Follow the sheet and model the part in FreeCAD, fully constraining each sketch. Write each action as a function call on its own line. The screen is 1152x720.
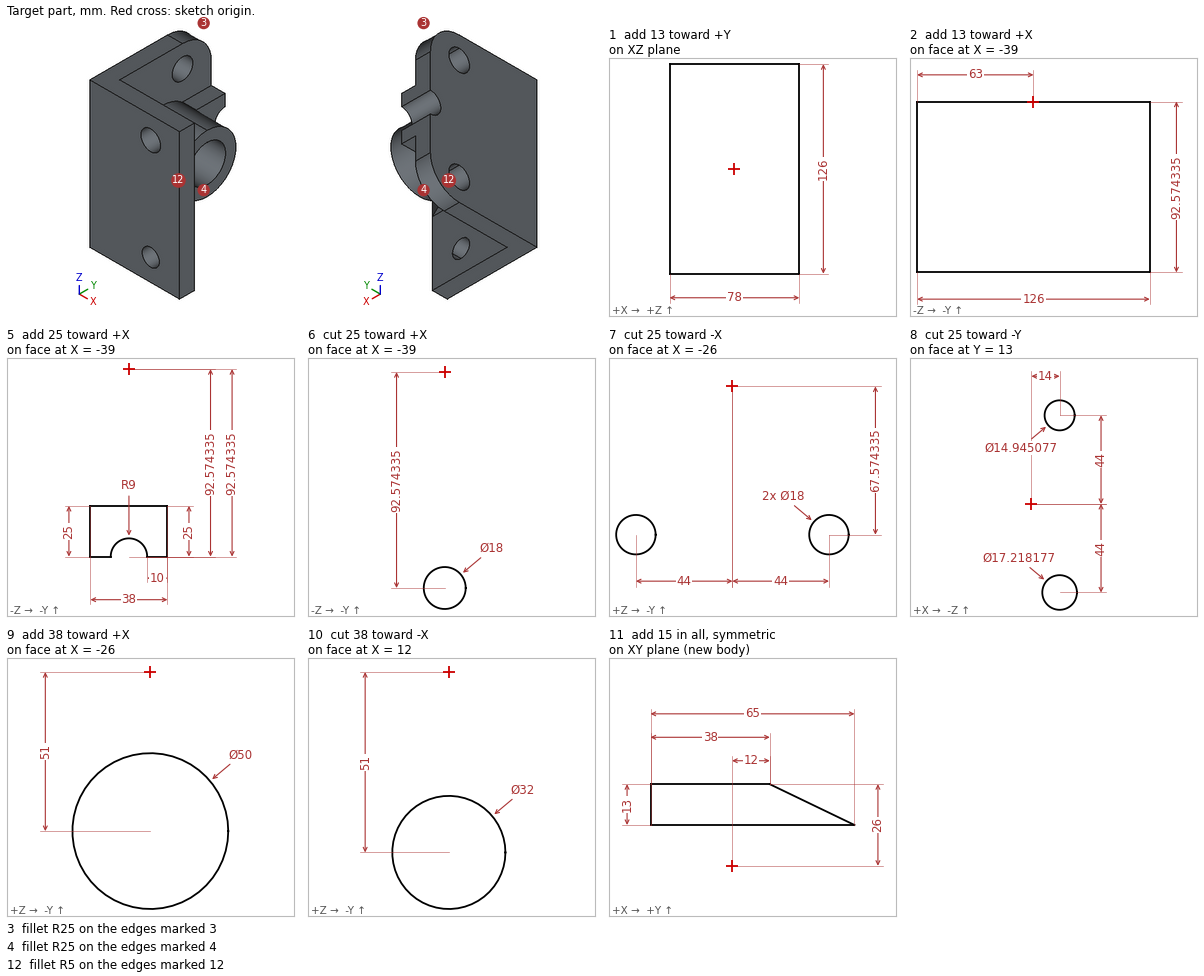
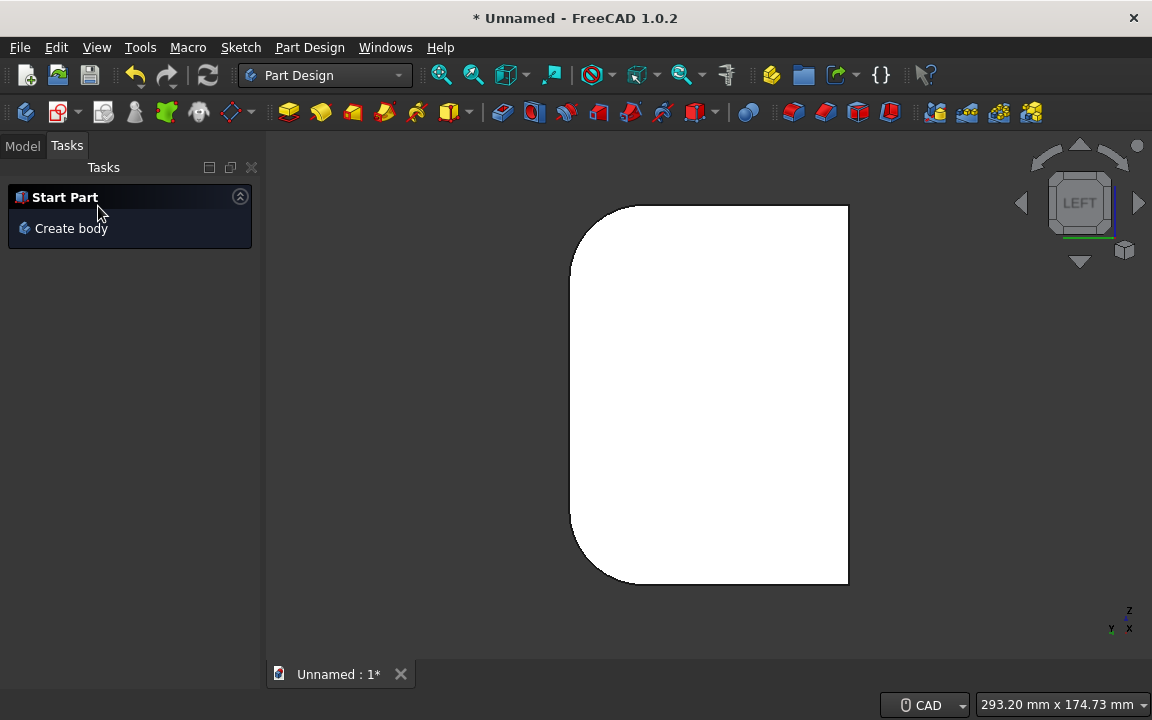
click(709, 394)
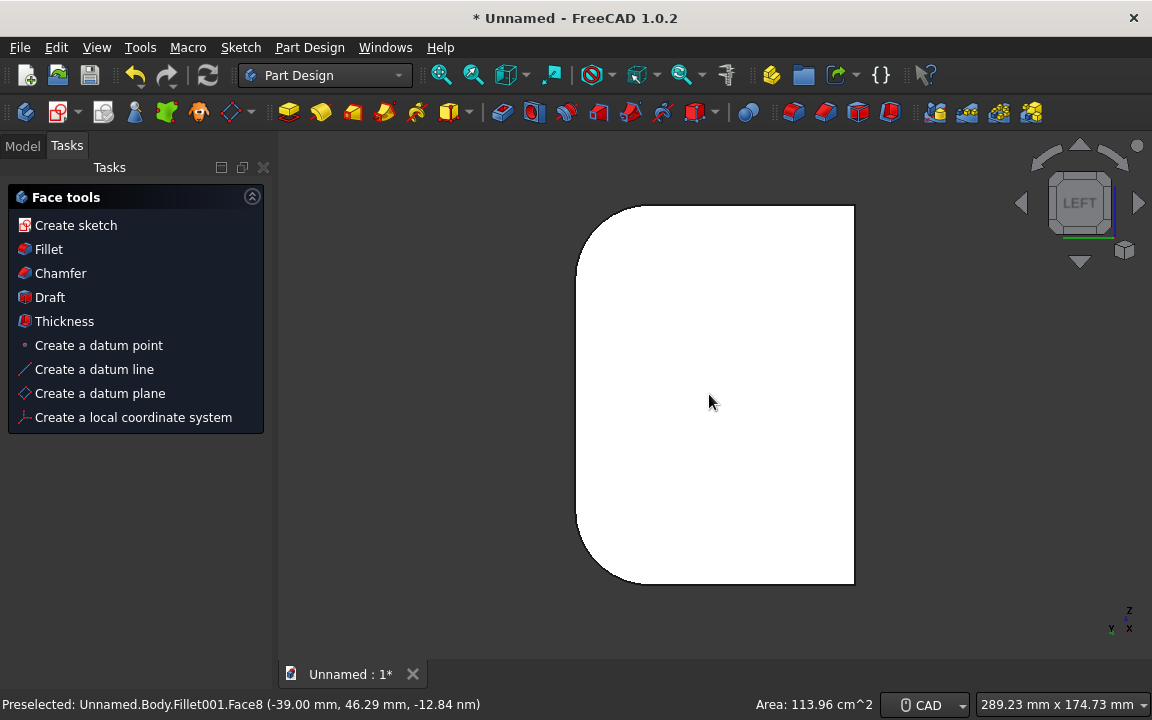
click(58, 112)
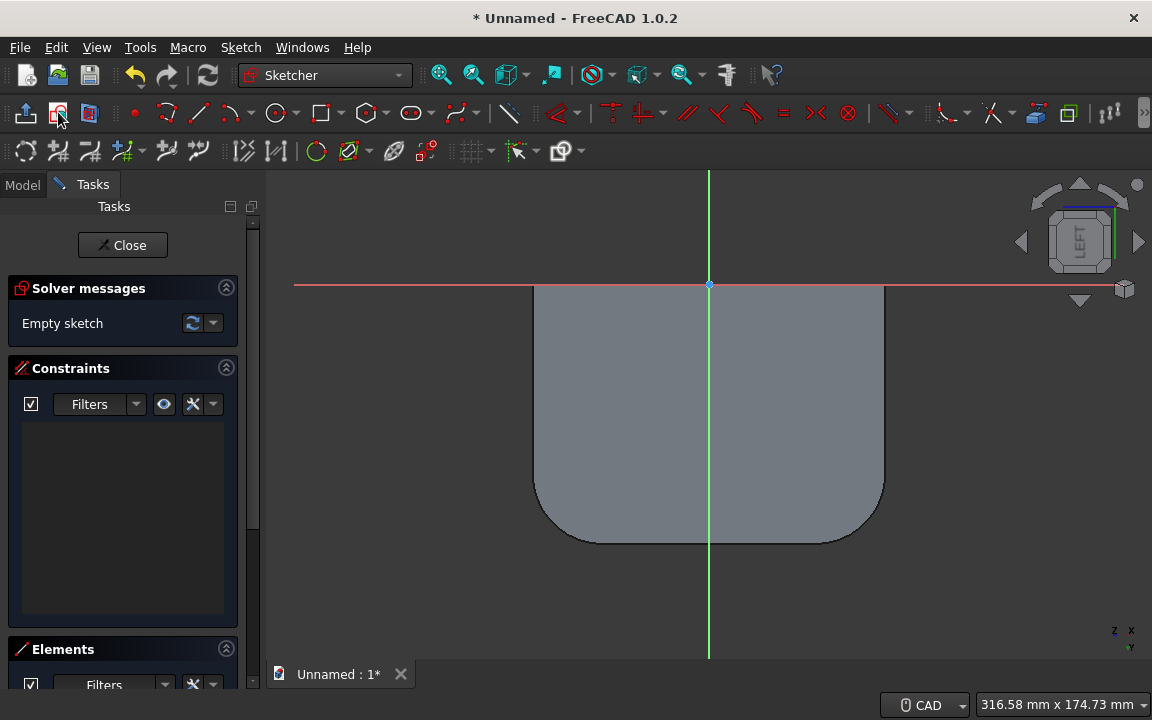
click(168, 114)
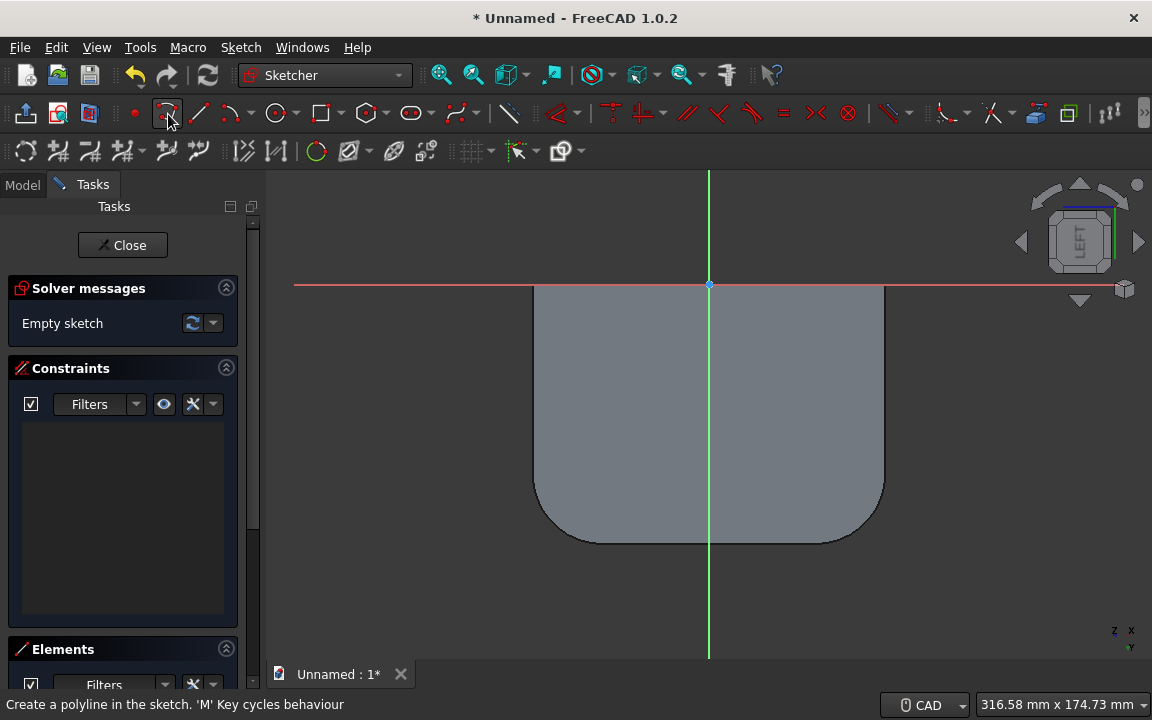
click(734, 544)
click(762, 544)
click(762, 474)
click(656, 474)
click(656, 544)
click(684, 544)
right_click(684, 544)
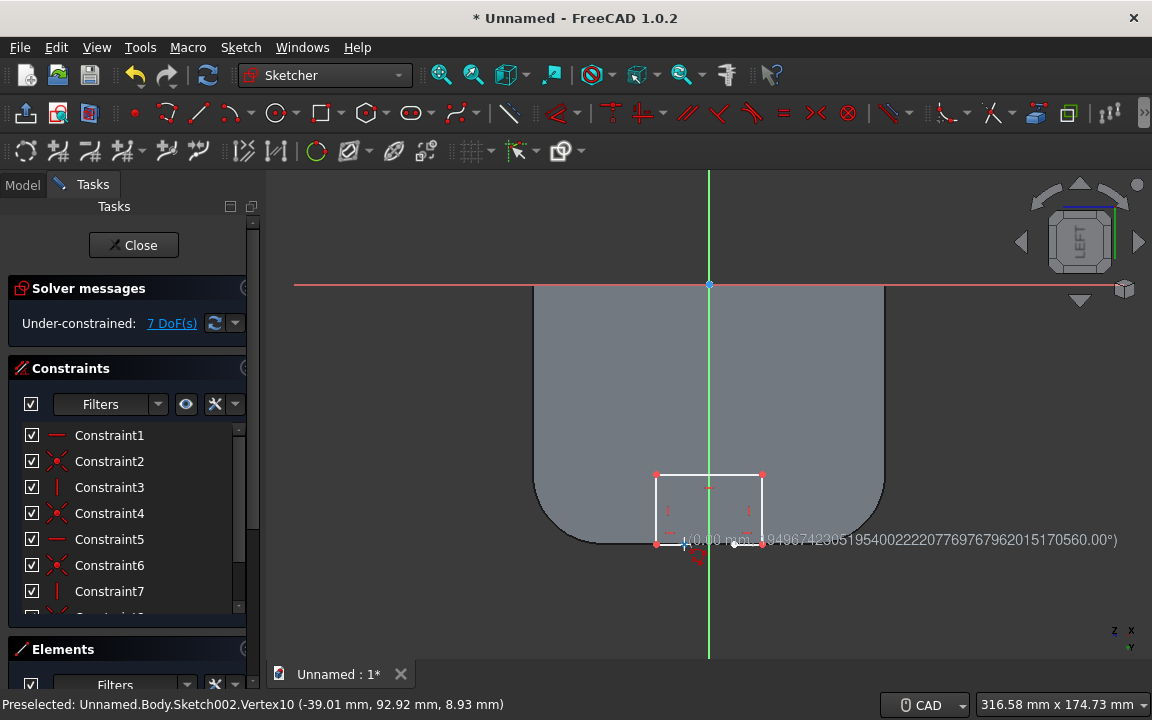
key(g)
key(3)
key(a)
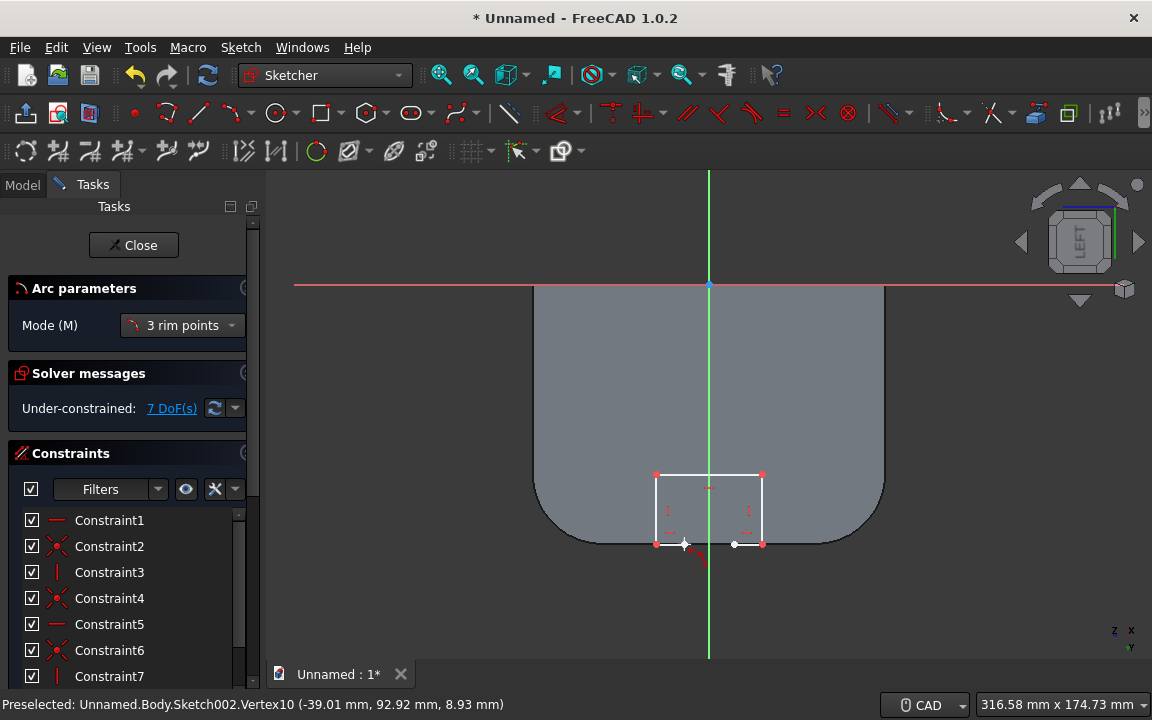
click(684, 545)
click(734, 545)
click(724, 524)
key(Escape)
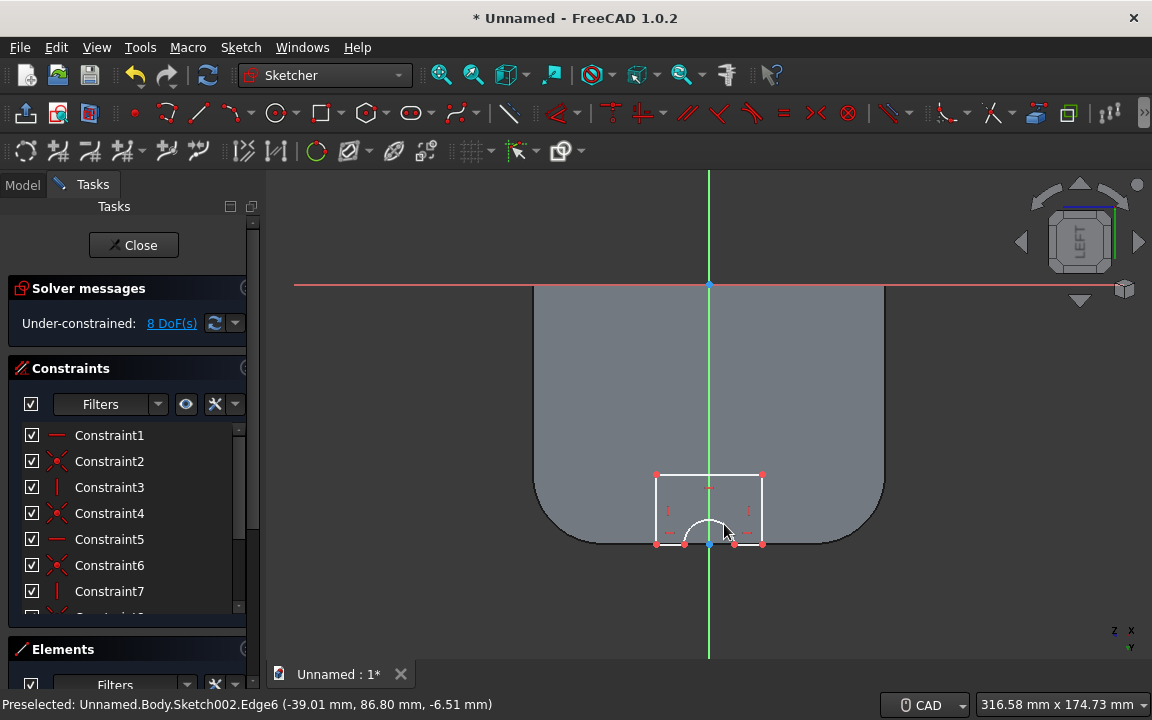
click(709, 545)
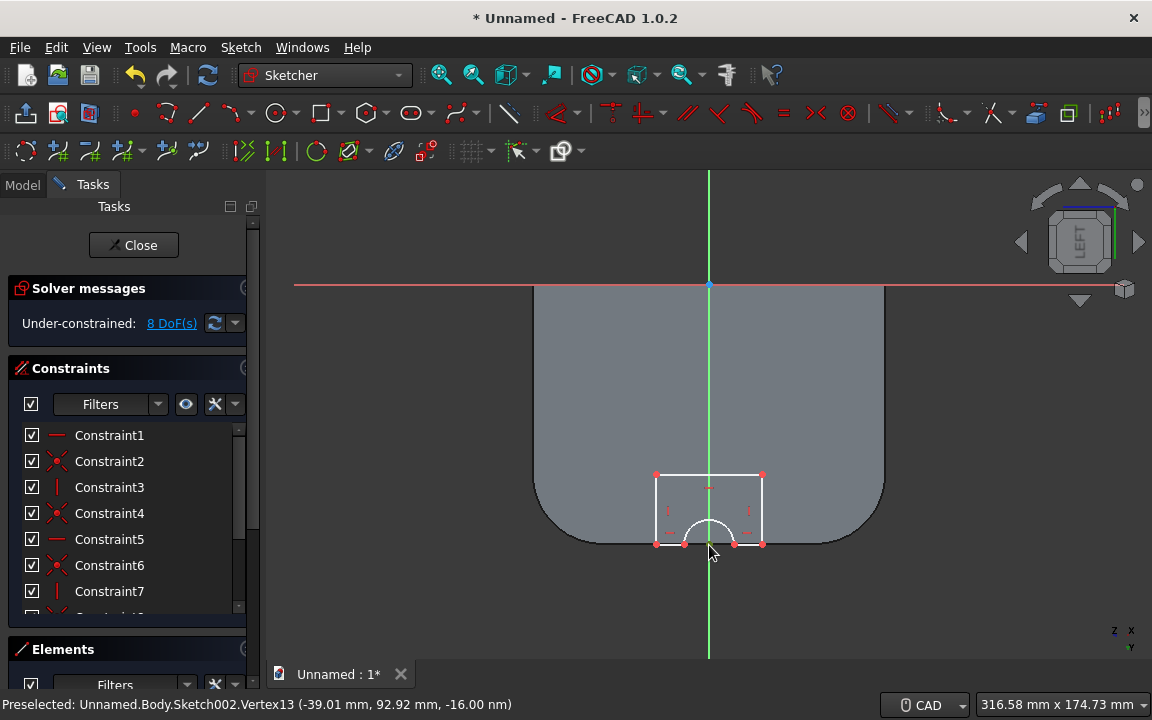
click(709, 600)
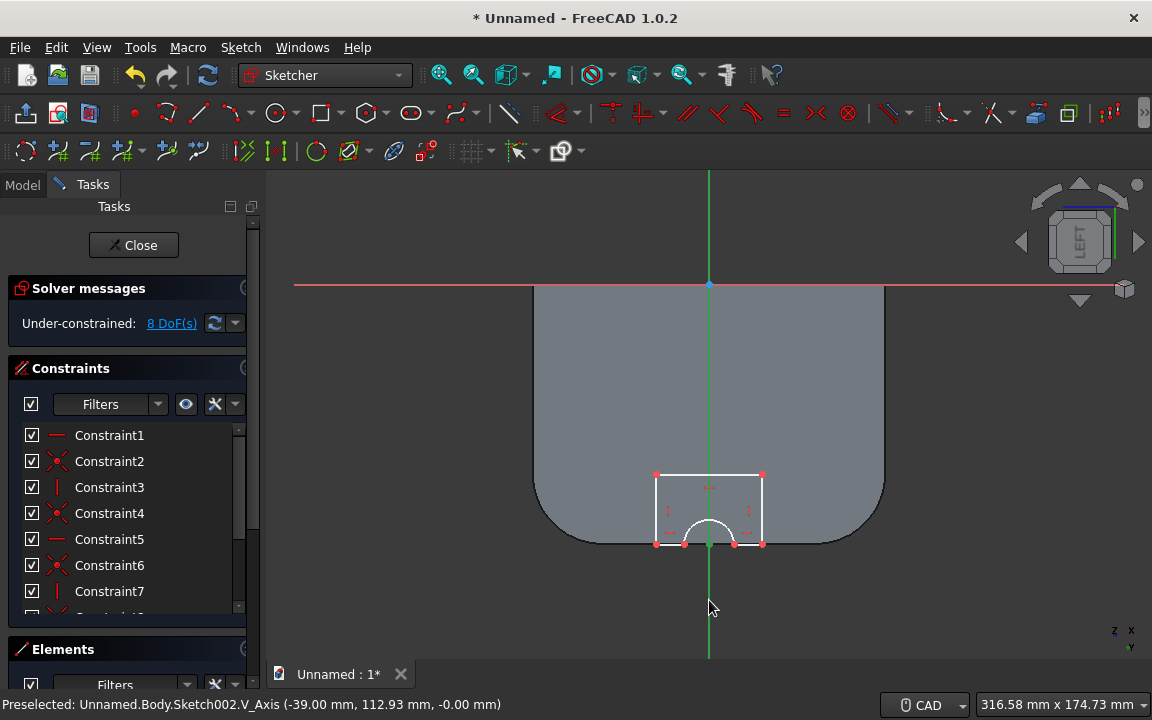
key(c)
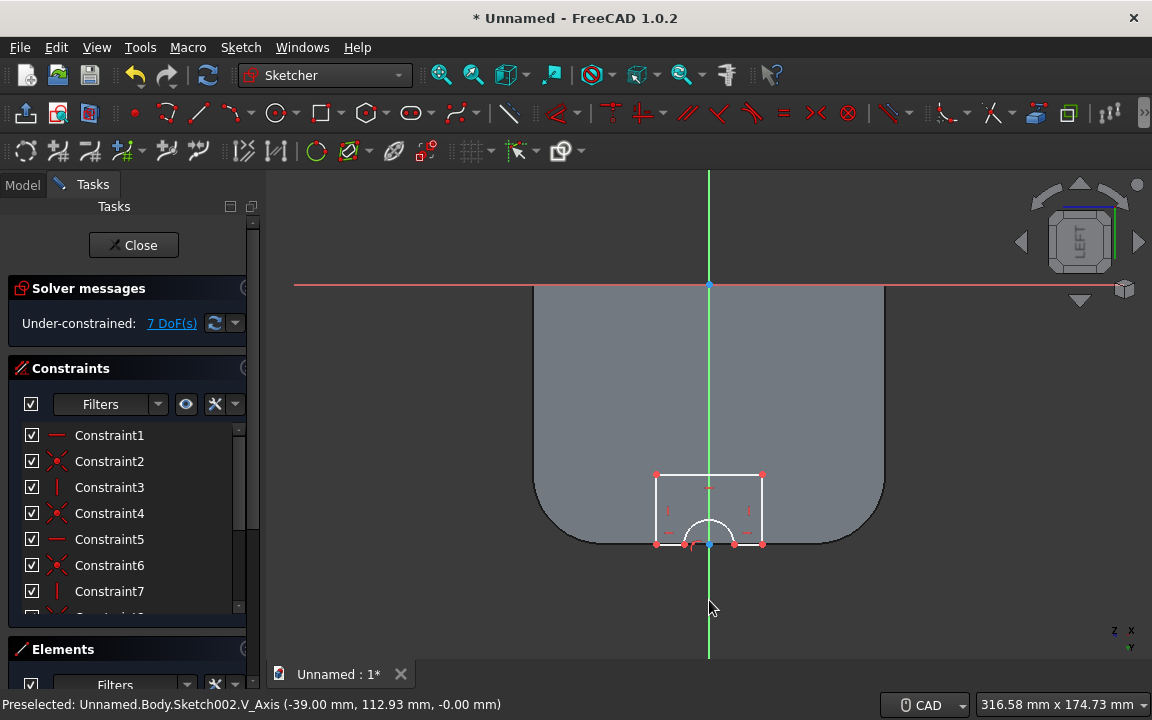
scroll(724, 525, up, 3)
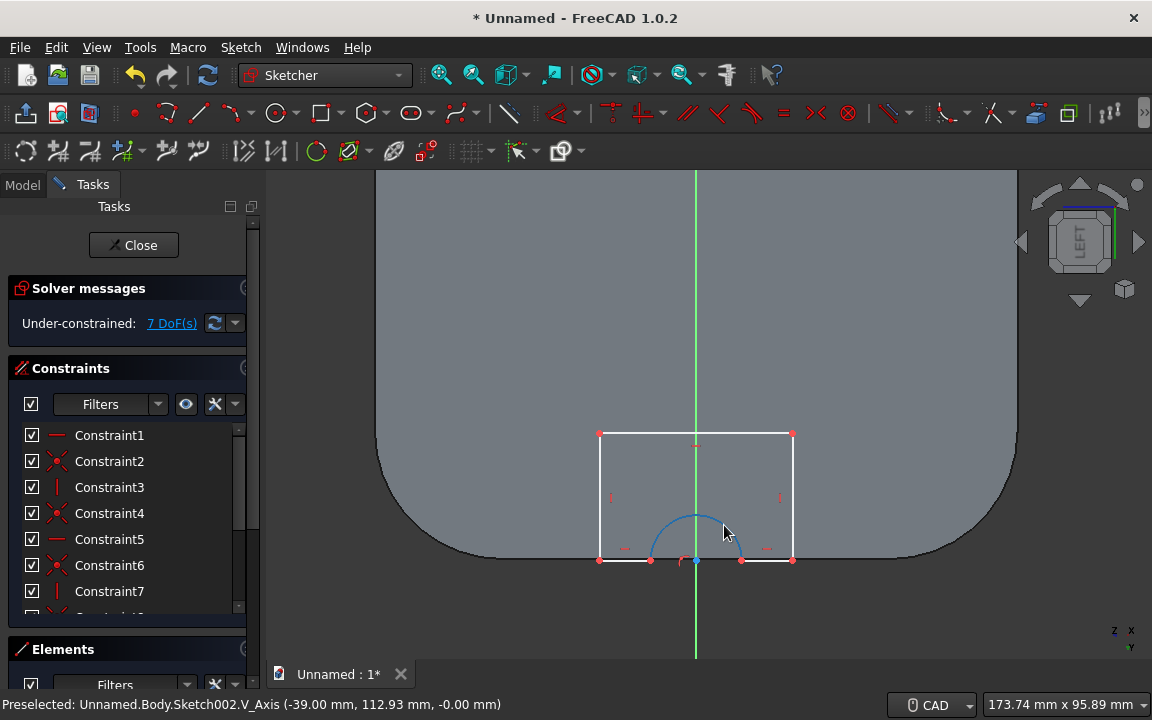
click(723, 524)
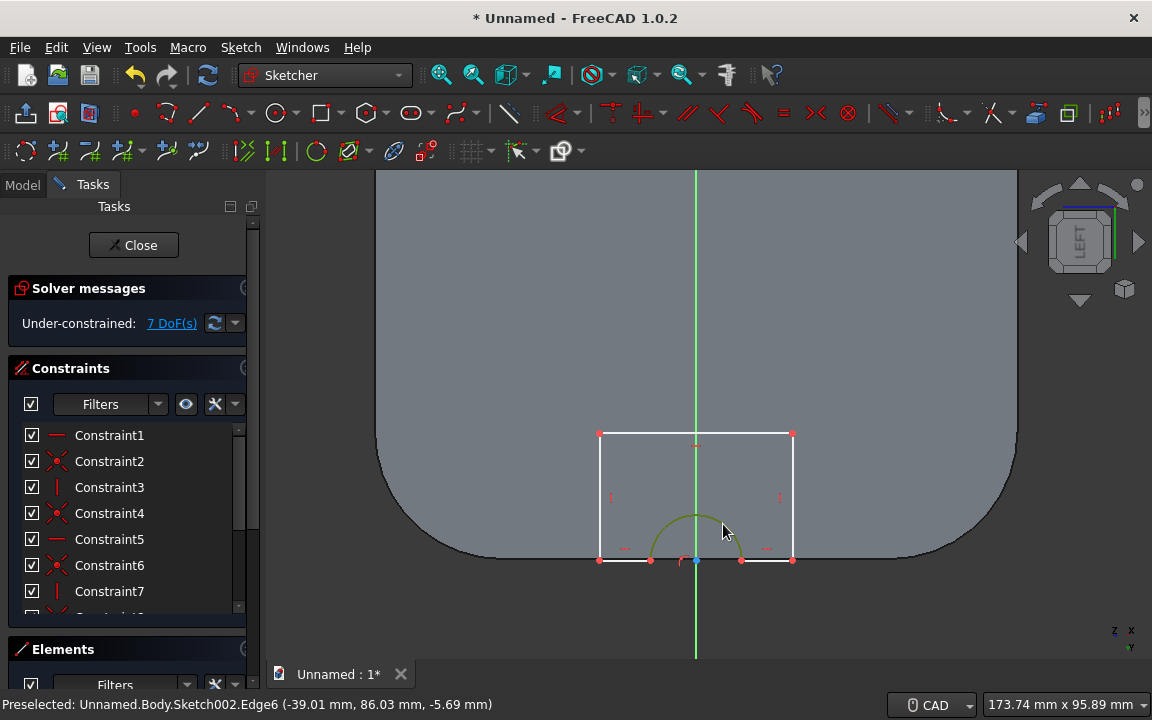
key(k)
key(r)